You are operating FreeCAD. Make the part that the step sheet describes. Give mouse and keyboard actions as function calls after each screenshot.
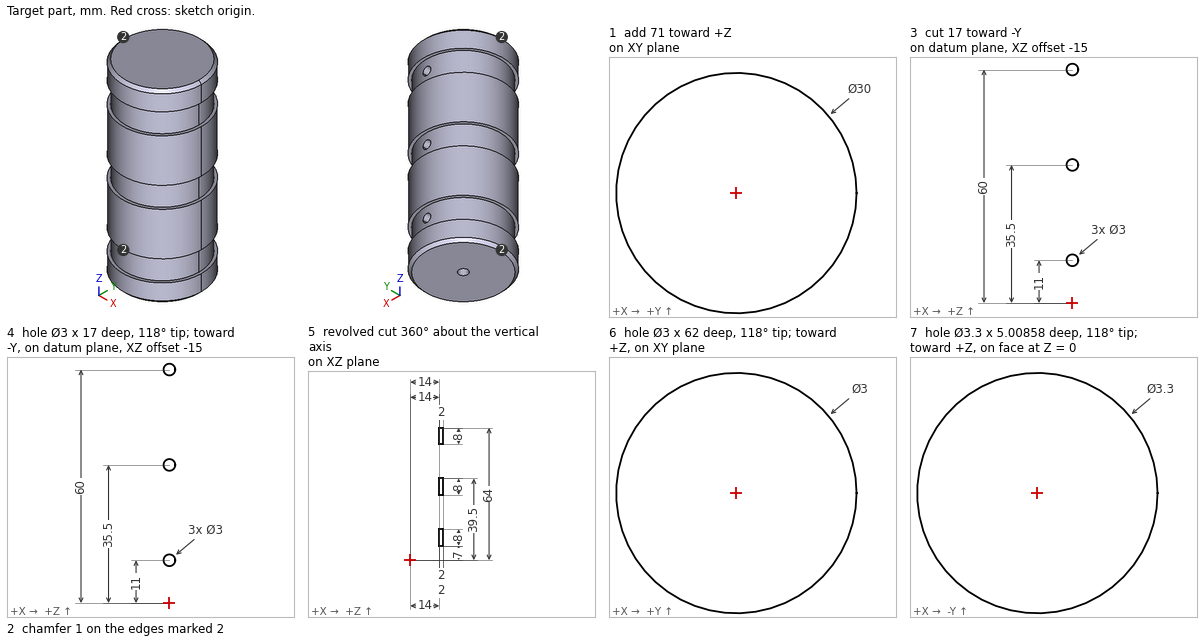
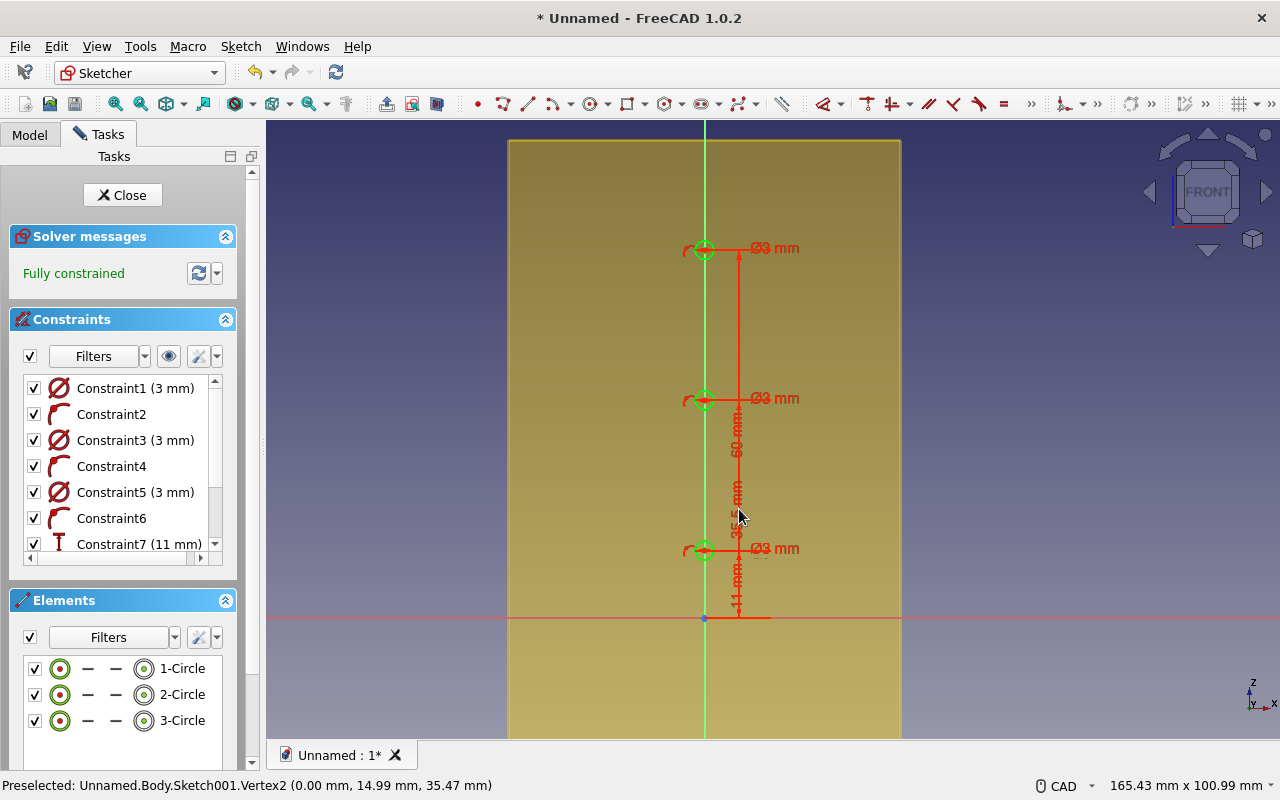
click(123, 195)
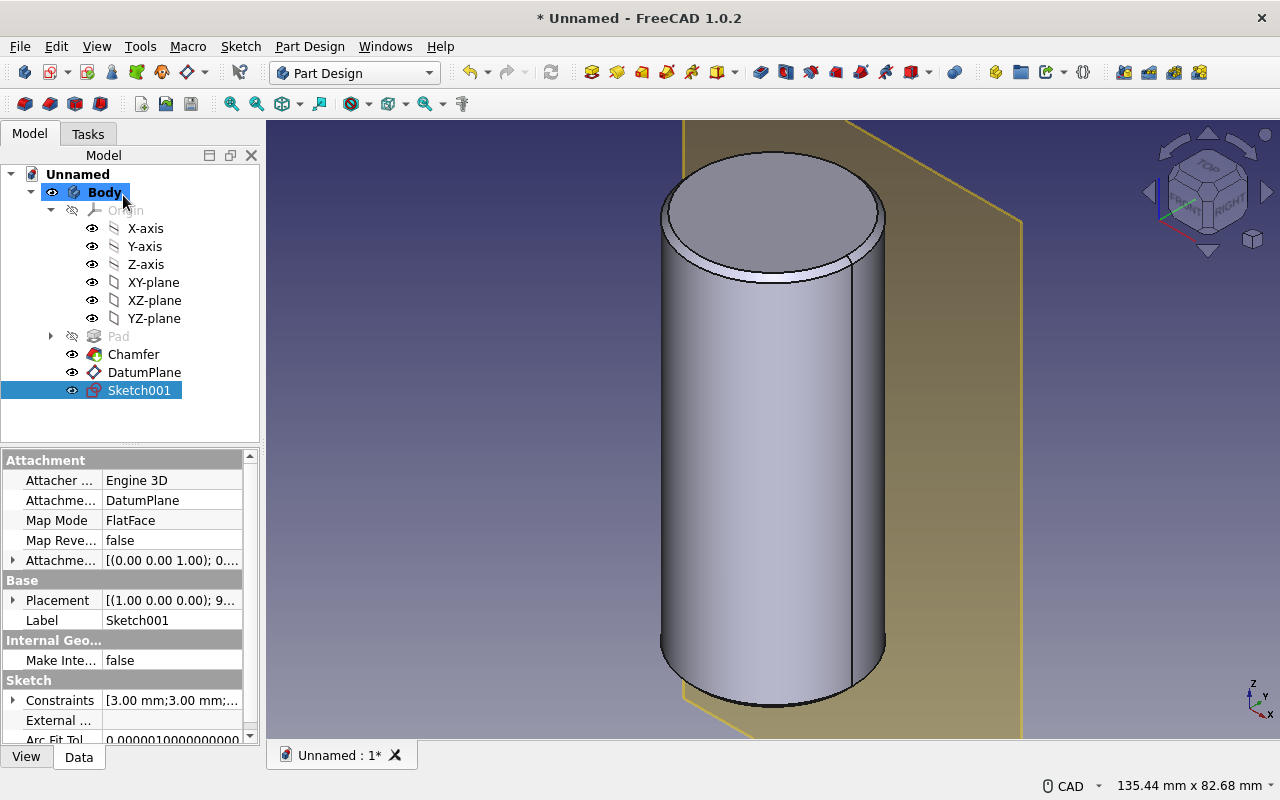
click(761, 72)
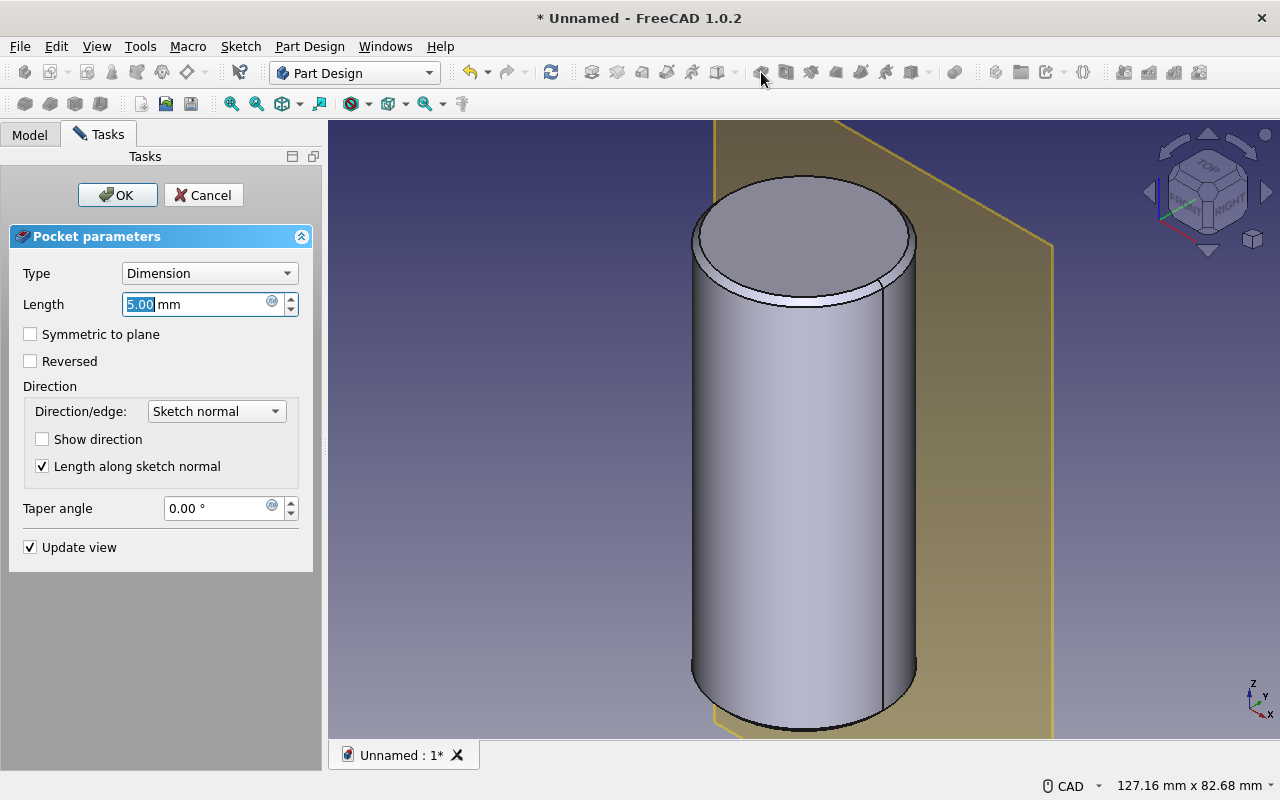
text(17)
key(Tab)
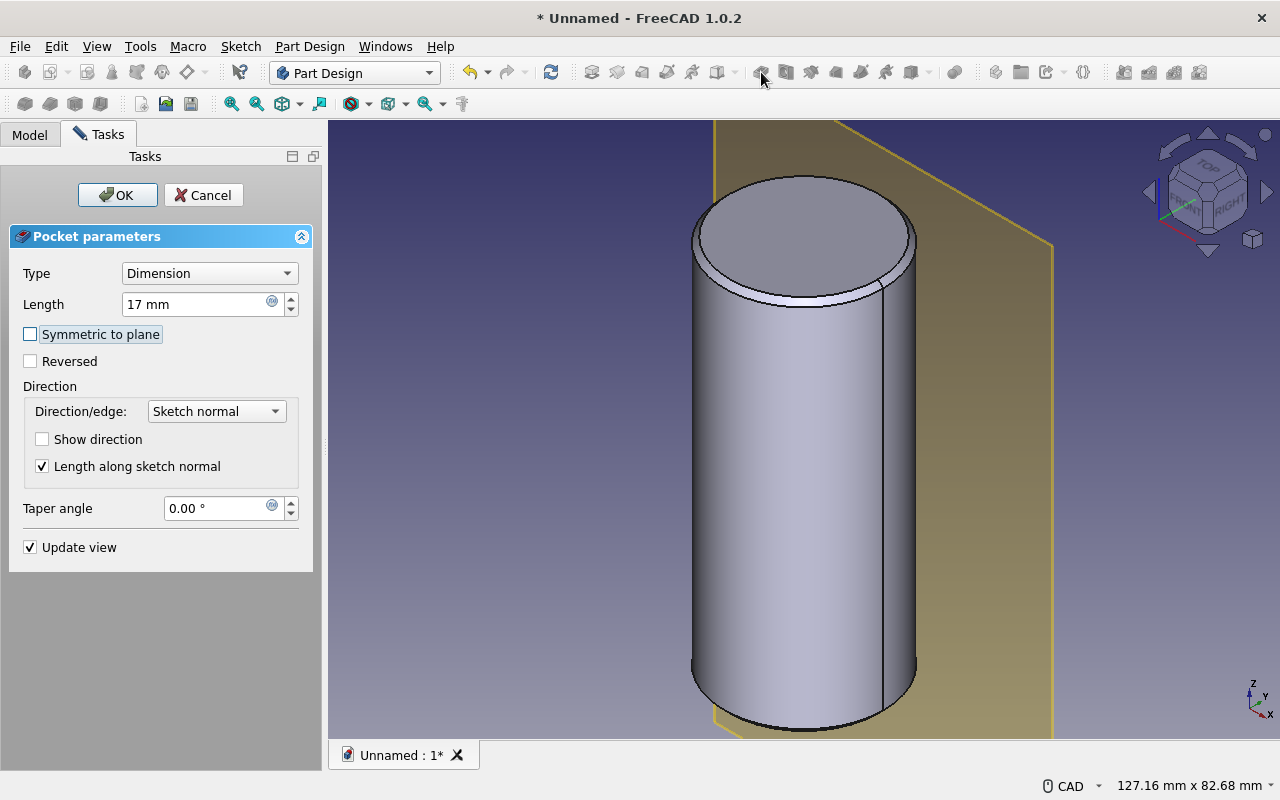
click(31, 361)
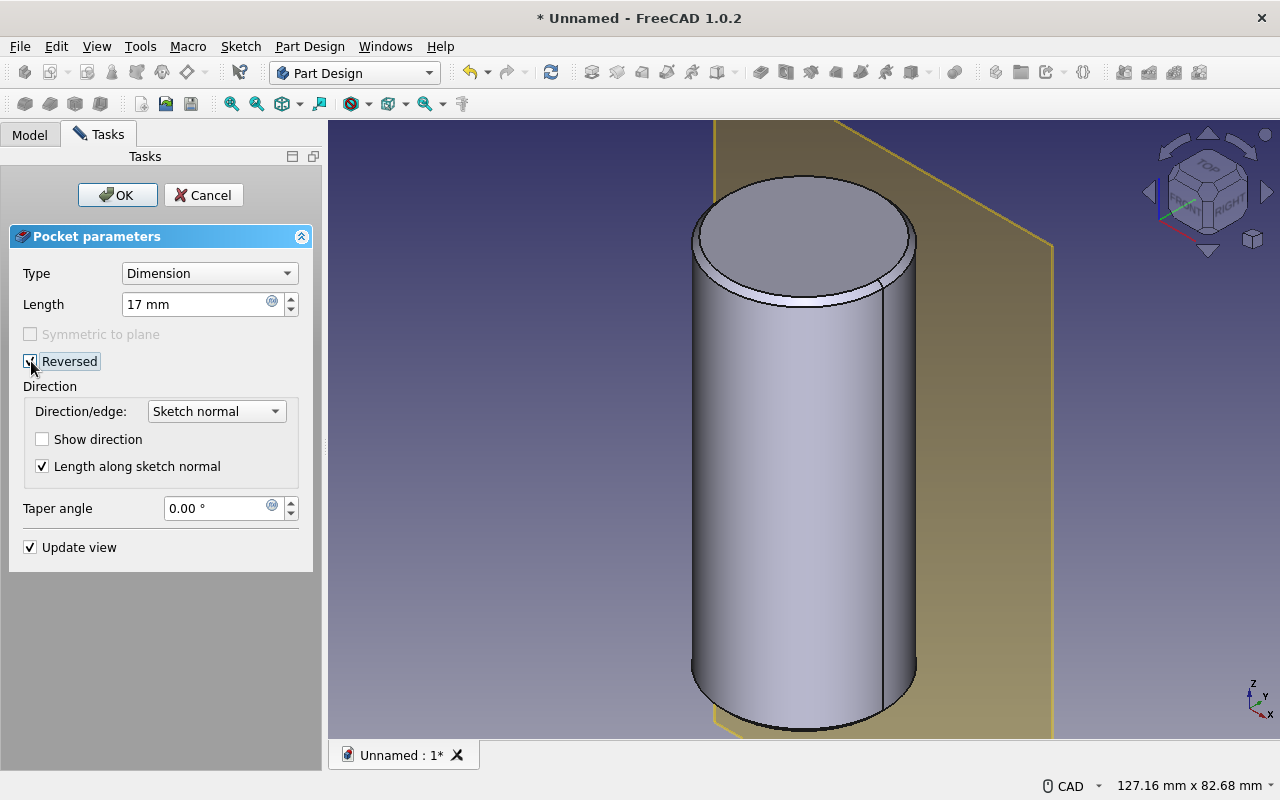
click(118, 195)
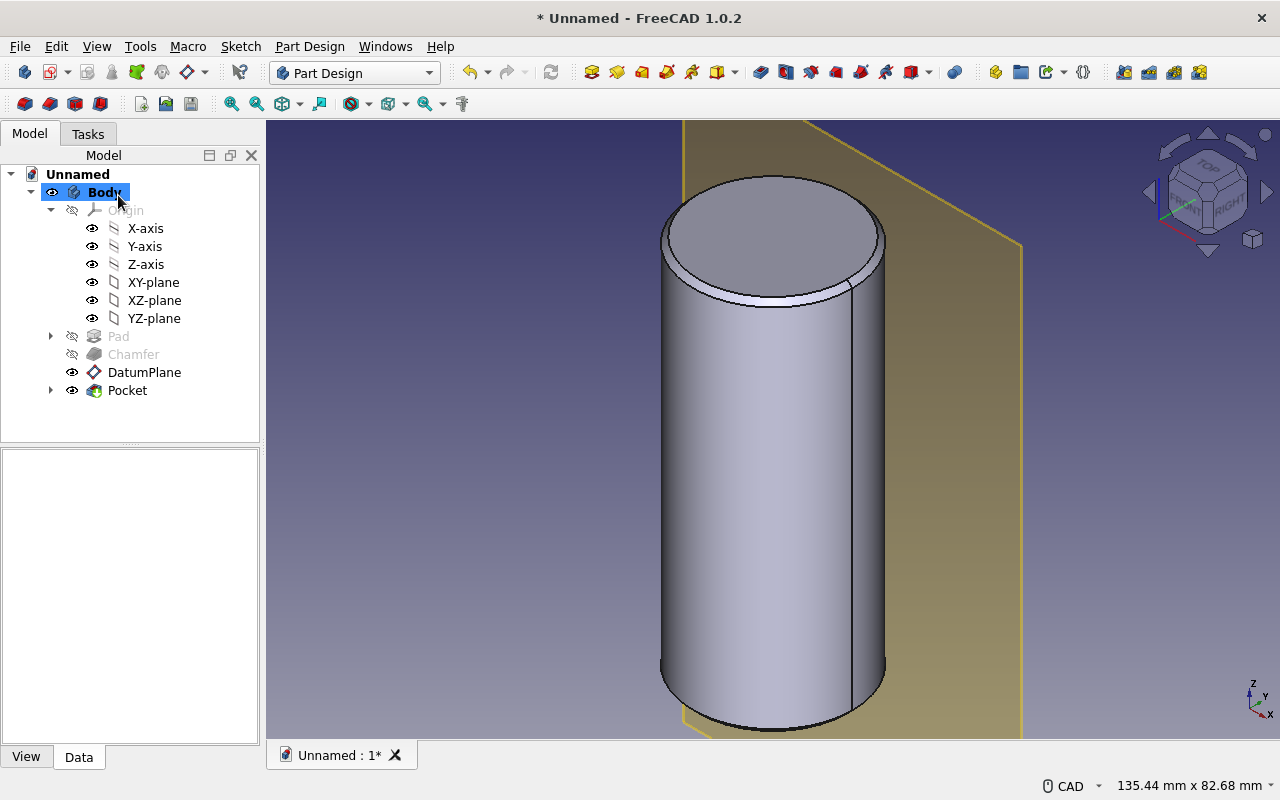
click(117, 372)
key(space)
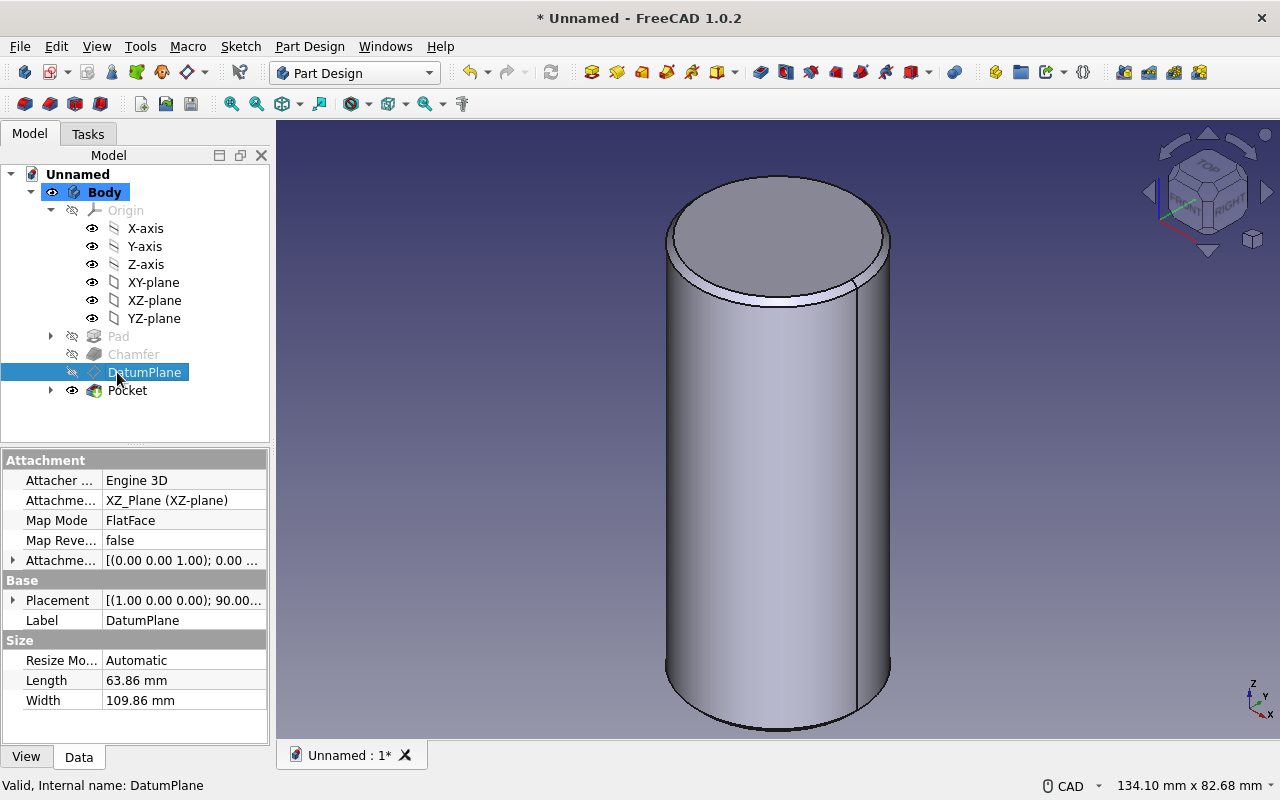
click(232, 104)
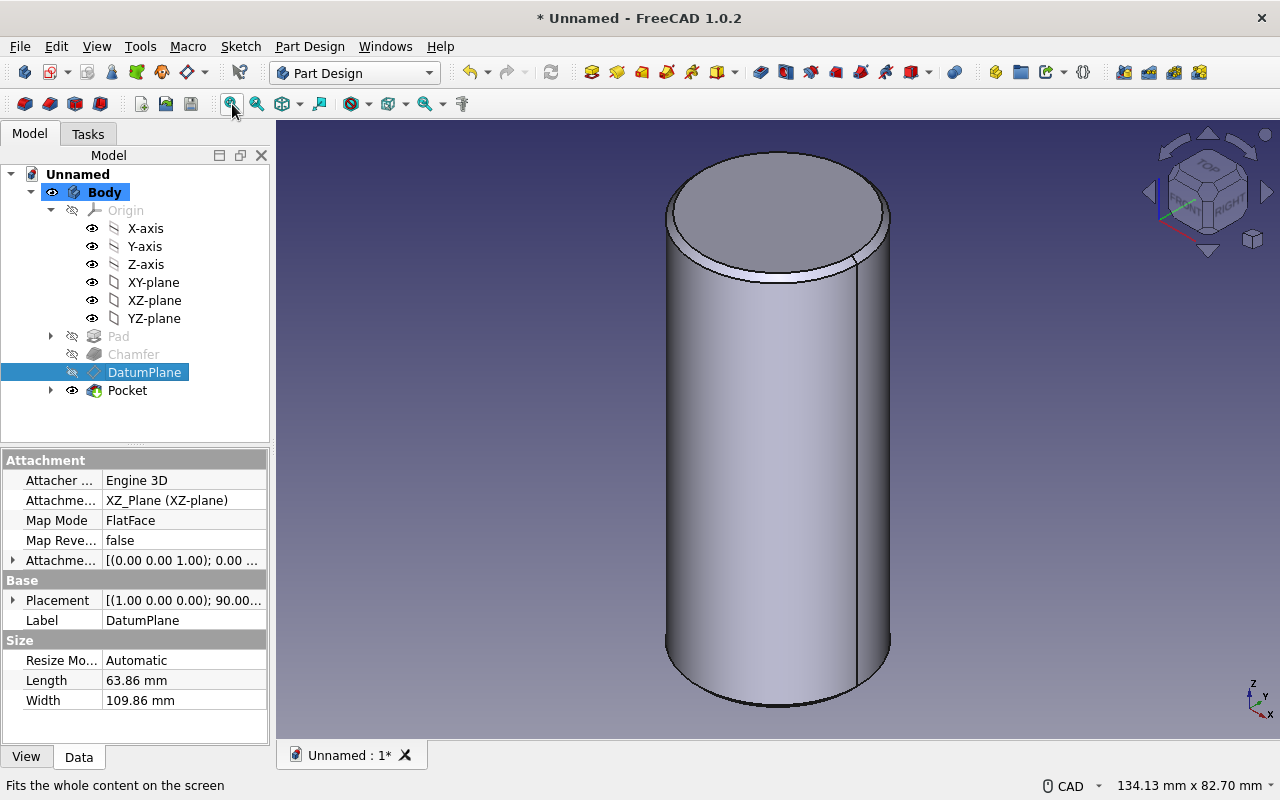
click(137, 300)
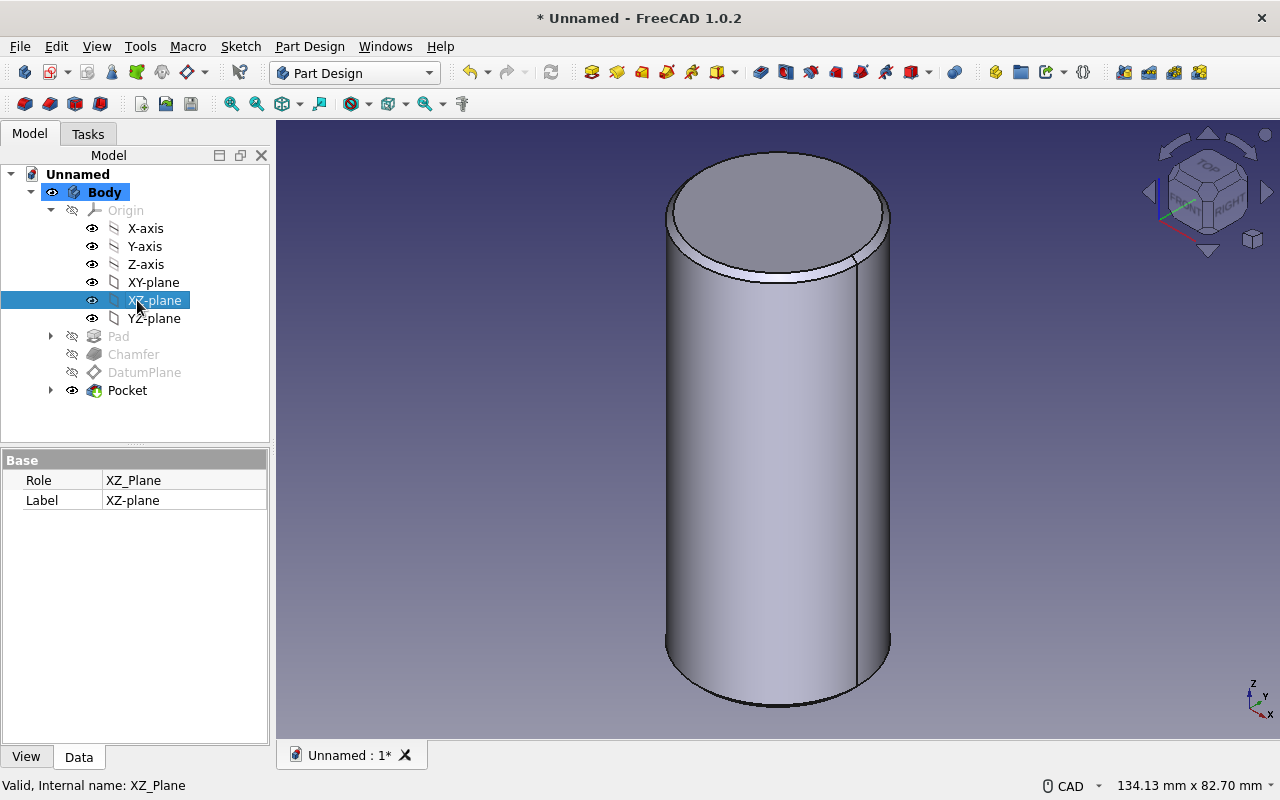
click(186, 72)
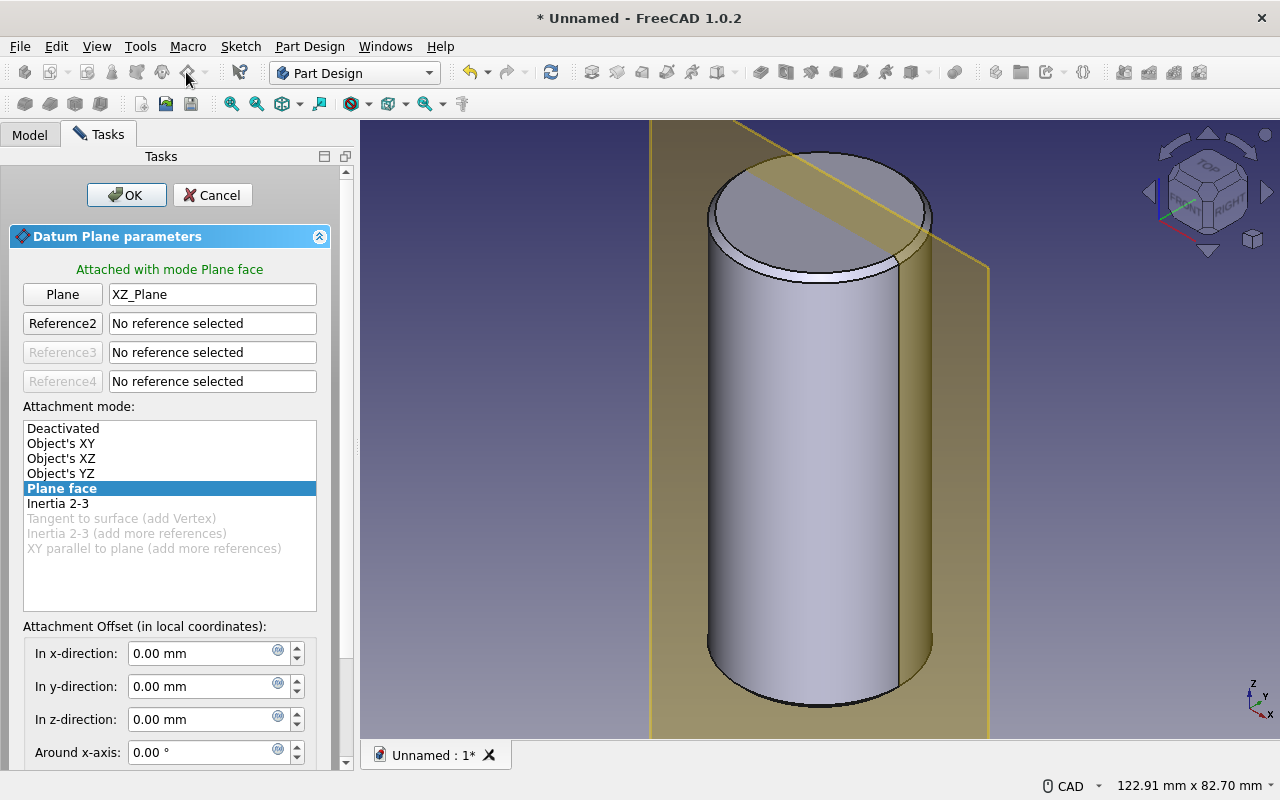
triple_click(210, 720)